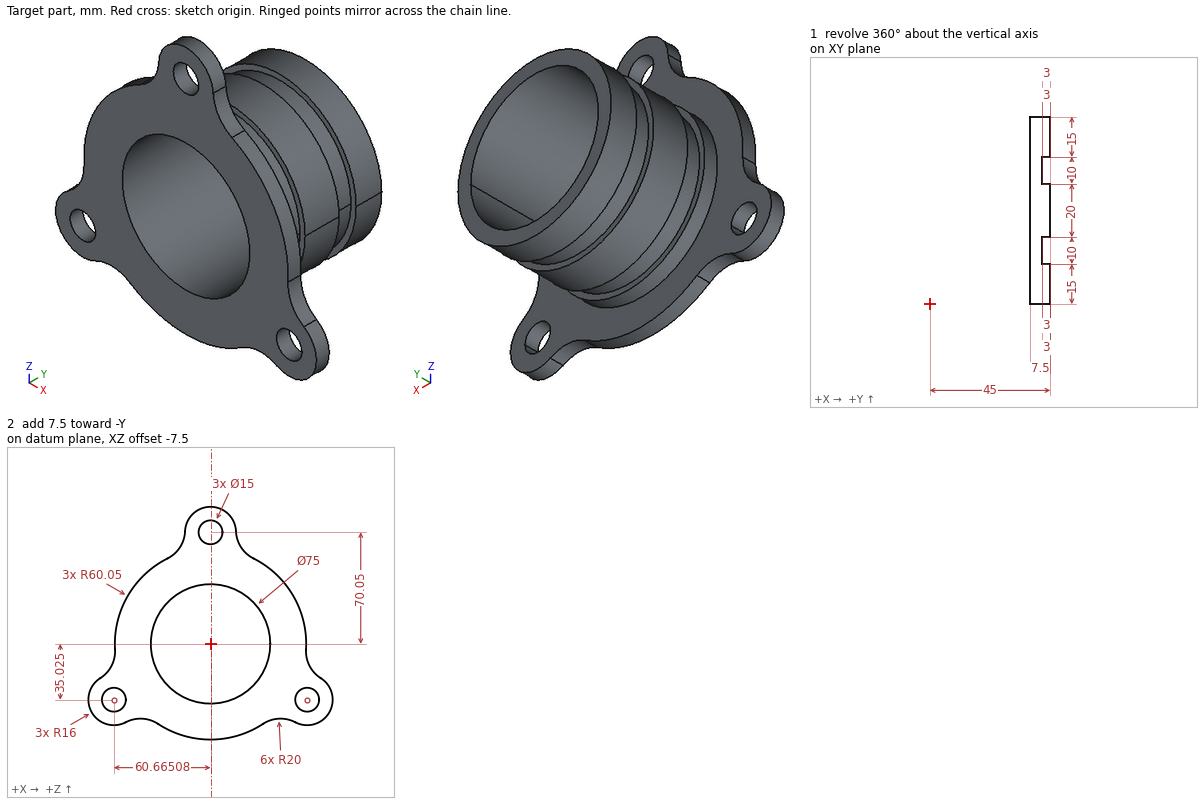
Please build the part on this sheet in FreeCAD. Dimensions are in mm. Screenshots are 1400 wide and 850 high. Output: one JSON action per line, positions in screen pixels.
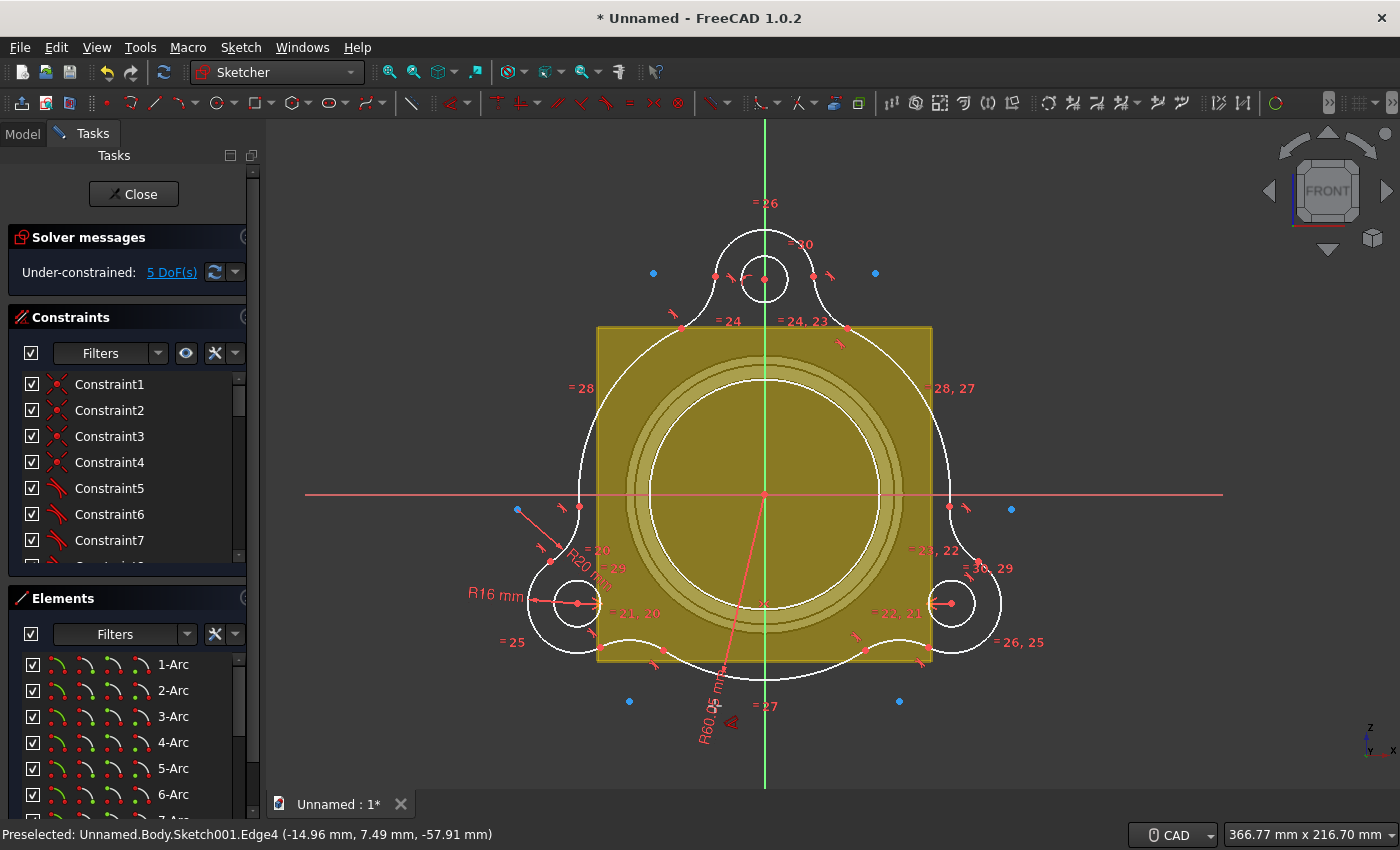
{"action": "left_click", "coordinate": [594, 587]}
{"action": "left_click", "coordinate": [632, 615]}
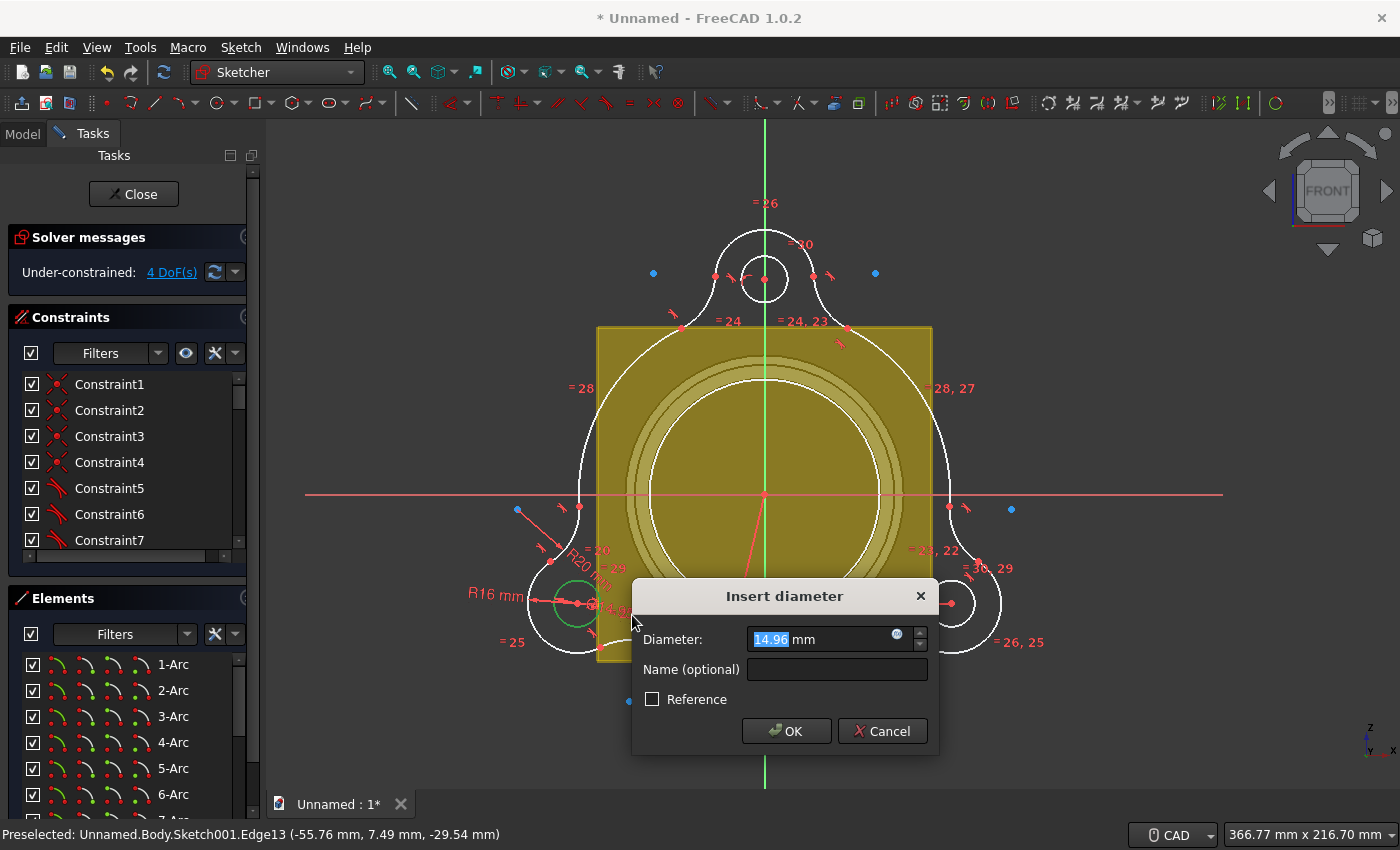
{"action": "type", "text": "15"}
{"action": "key", "text": "Return"}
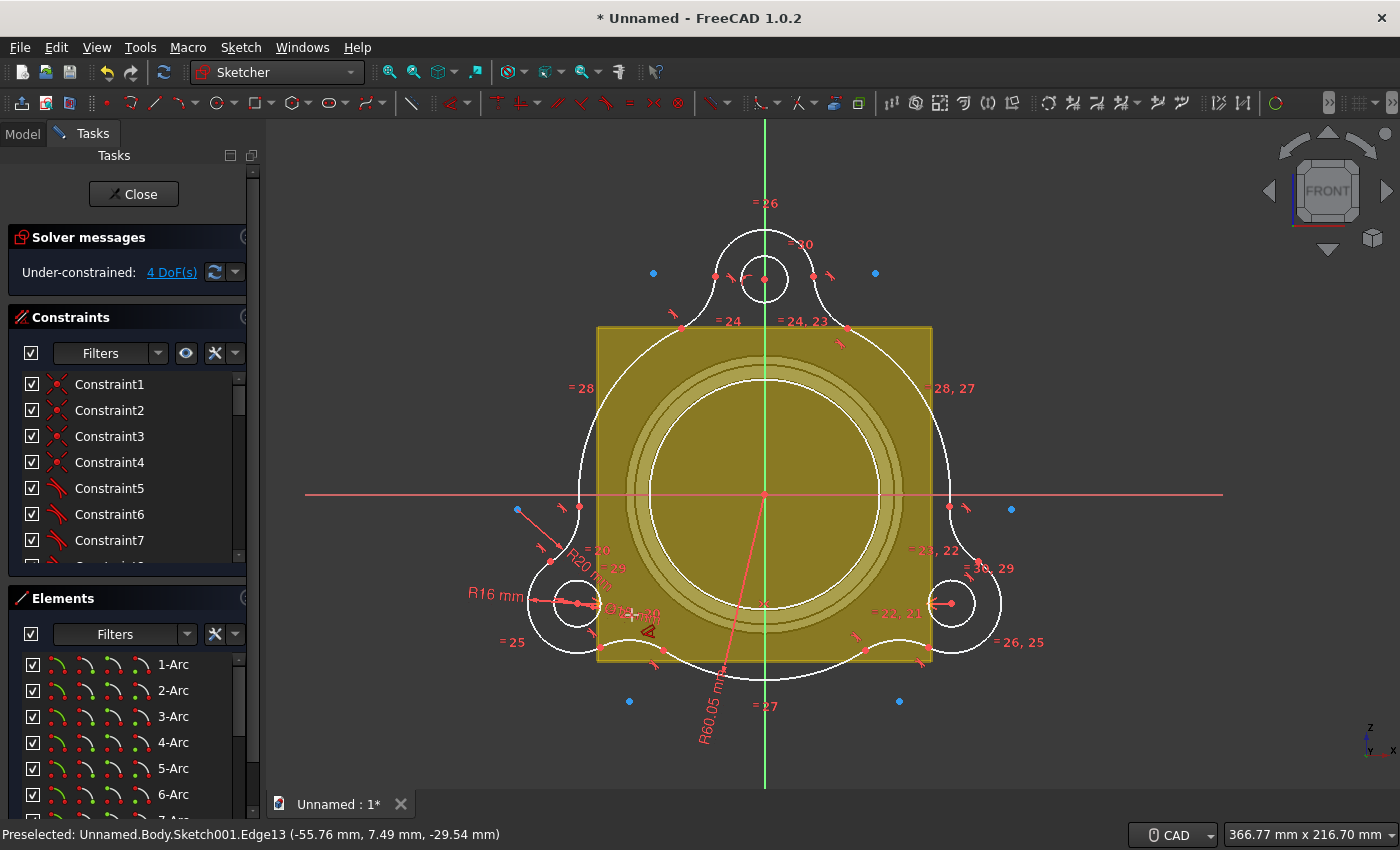
{"action": "left_click", "coordinate": [846, 413]}
{"action": "left_click", "coordinate": [869, 390]}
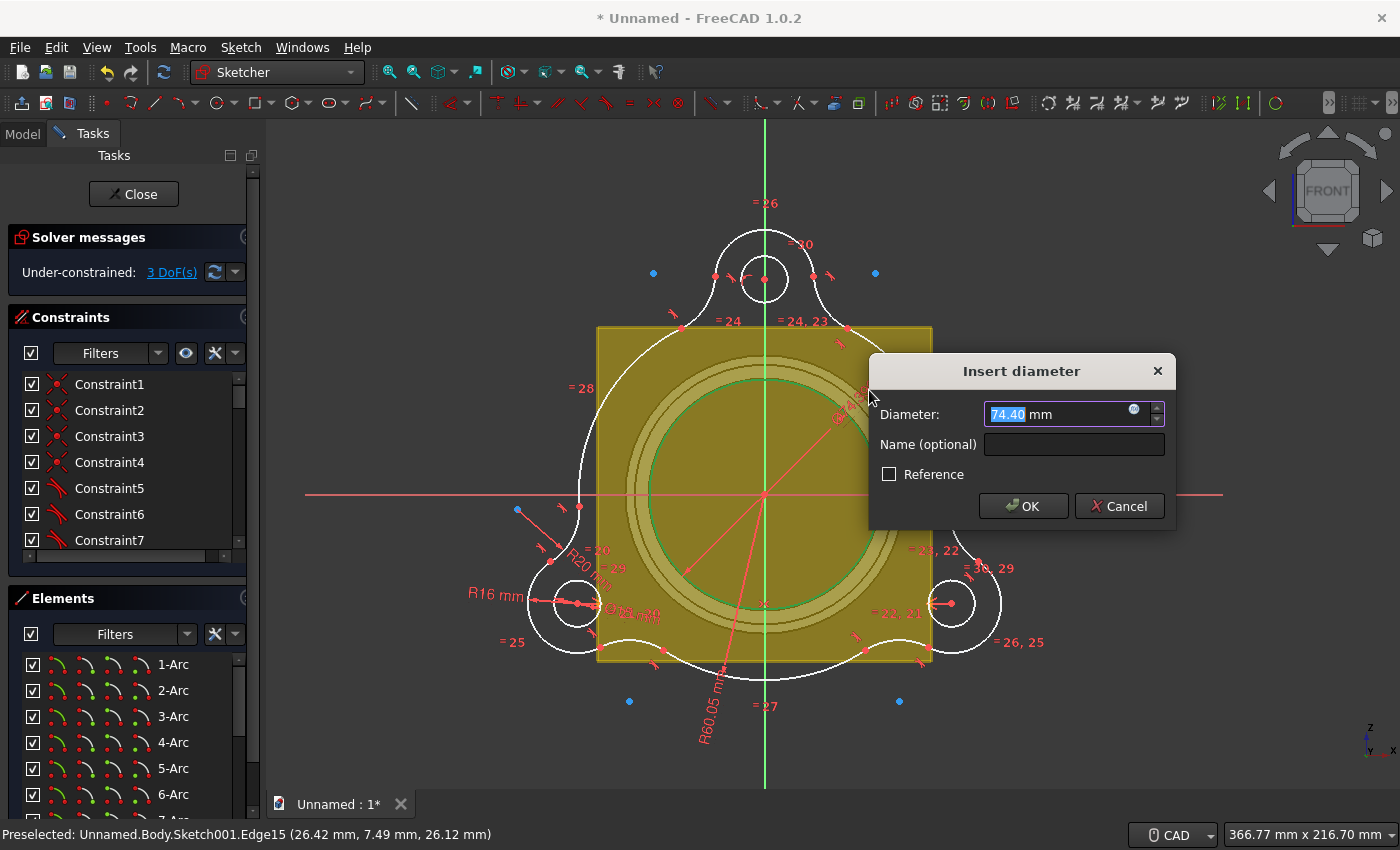
{"action": "type", "text": "75"}
{"action": "key", "text": "Return"}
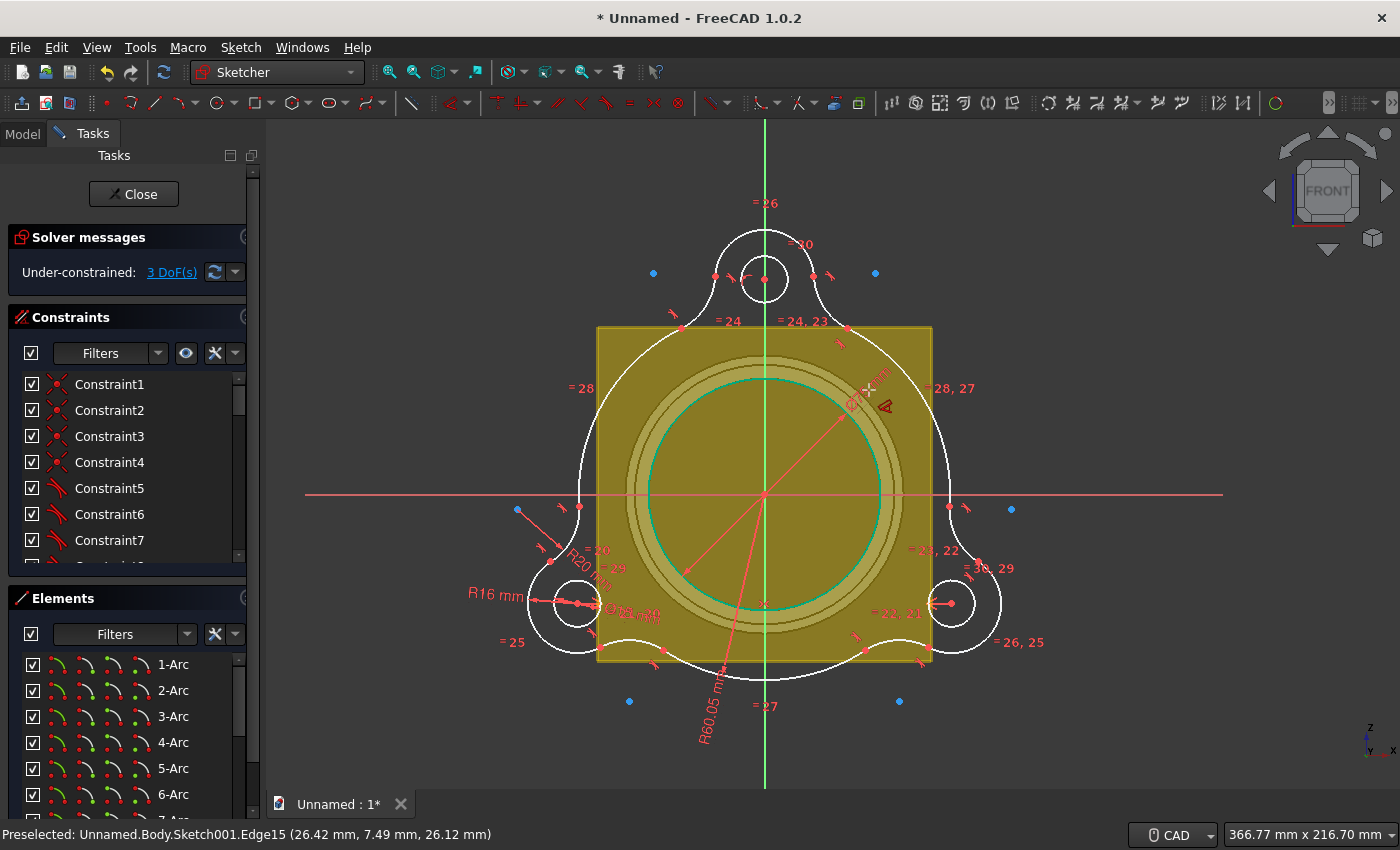
{"action": "left_click", "coordinate": [765, 279]}
{"action": "left_click", "coordinate": [799, 337]}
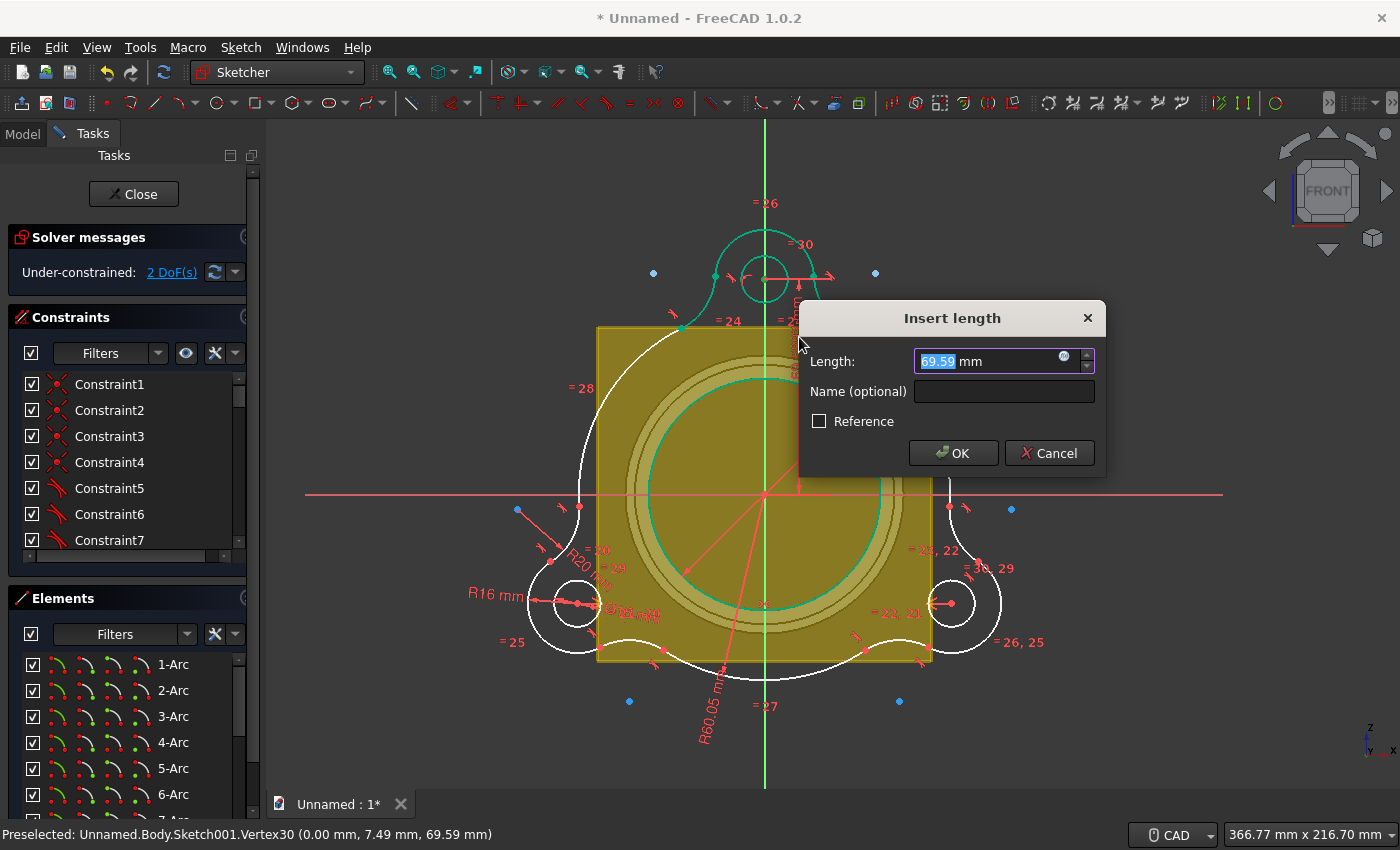
{"action": "type", "text": "70.05"}
{"action": "key", "text": "Return"}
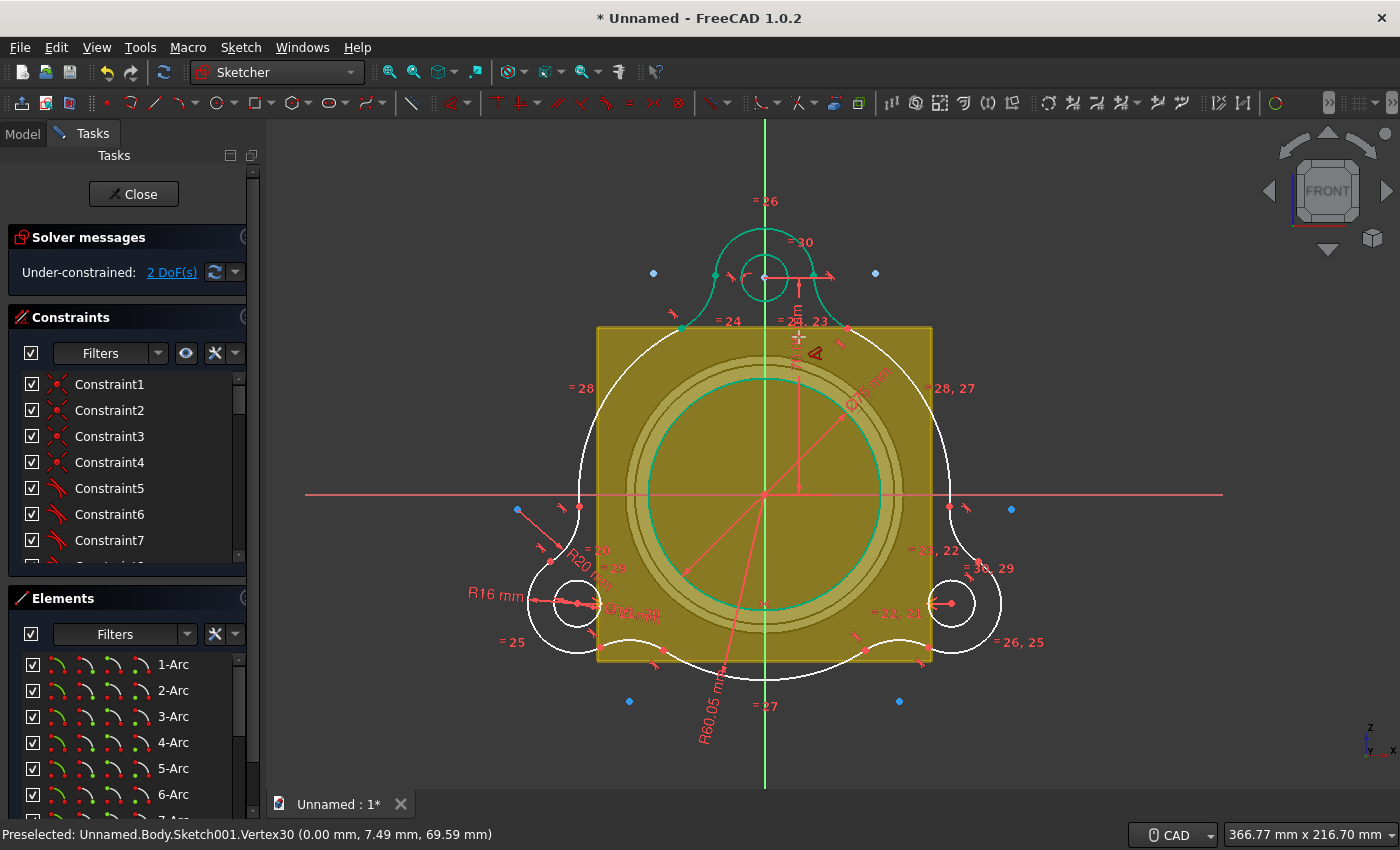
{"action": "left_click", "coordinate": [577, 604]}
{"action": "left_click", "coordinate": [543, 524]}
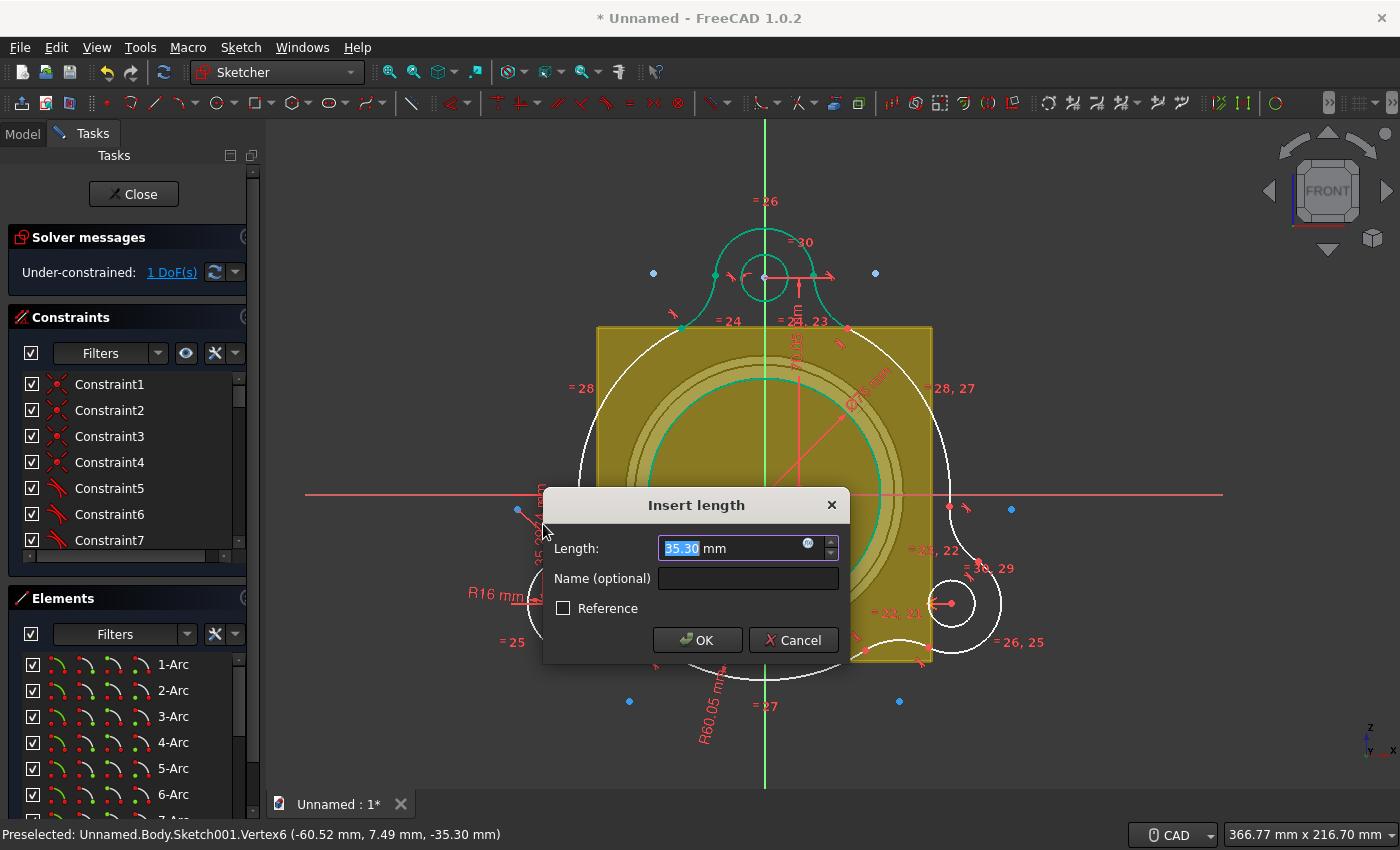
{"action": "type", "text": "35.025"}
{"action": "key", "text": "Return"}